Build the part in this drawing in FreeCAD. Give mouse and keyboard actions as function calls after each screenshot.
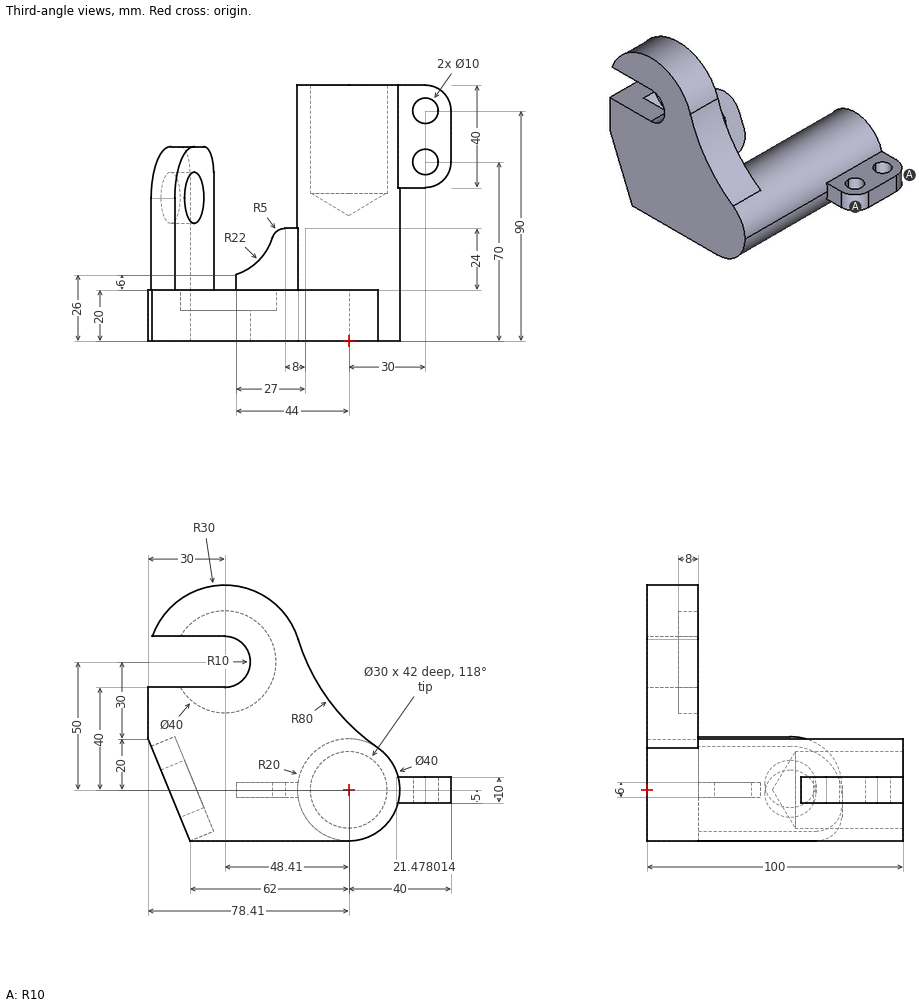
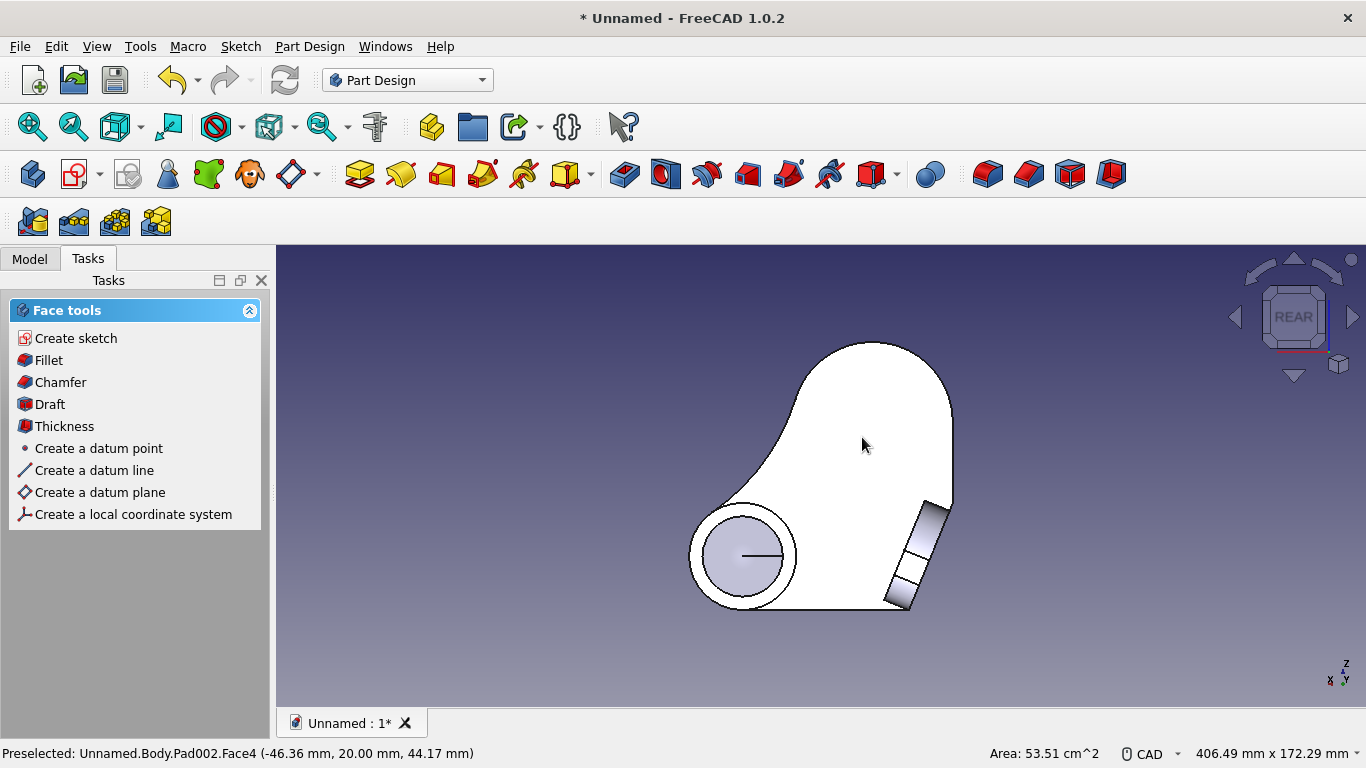
click(74, 174)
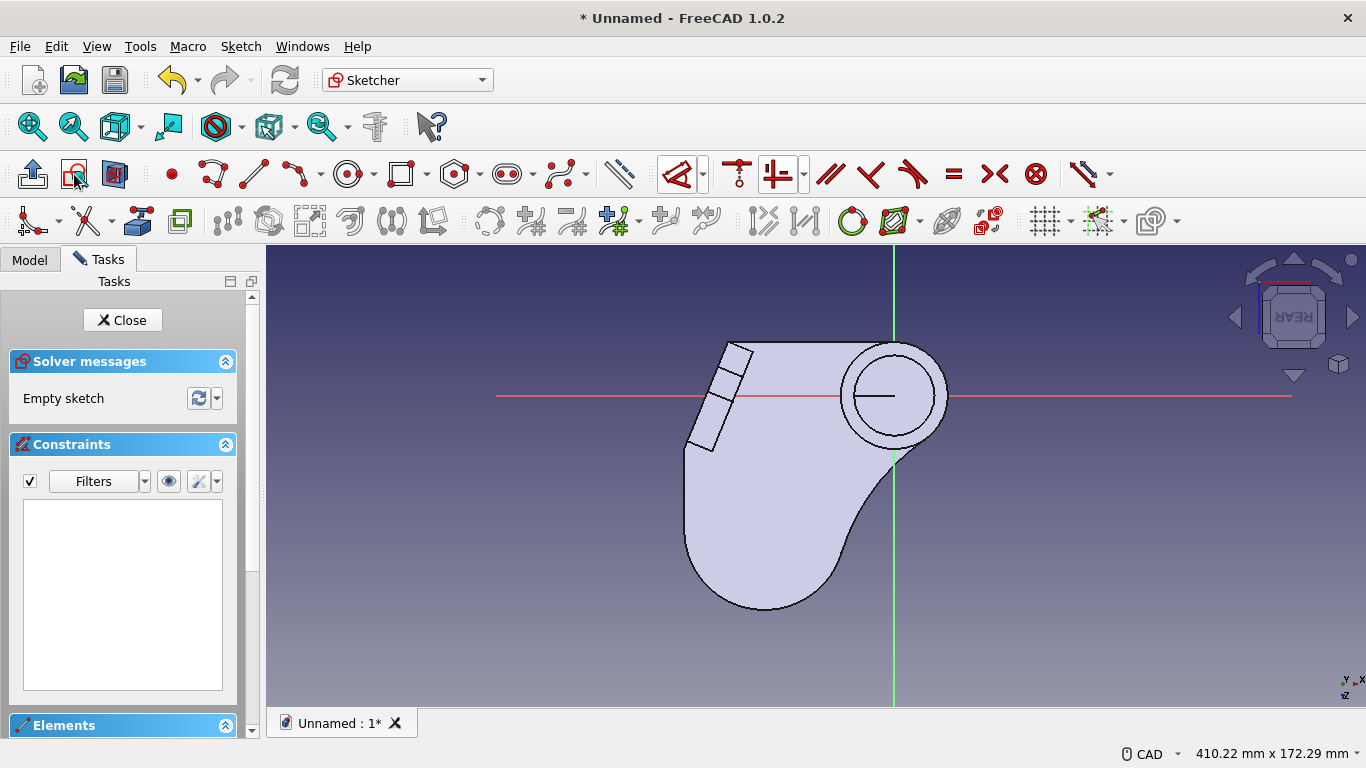
scroll(840, 476, up, 3)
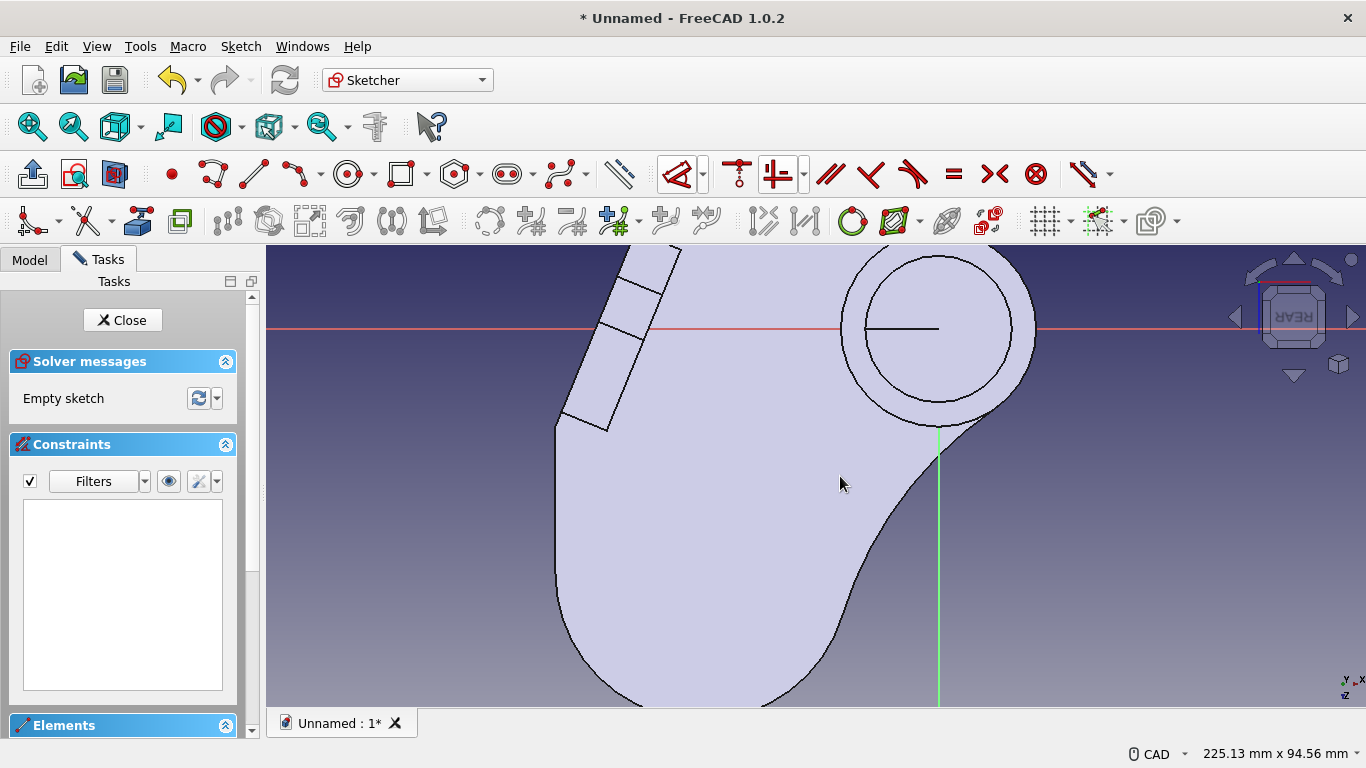
key(g)
key(m)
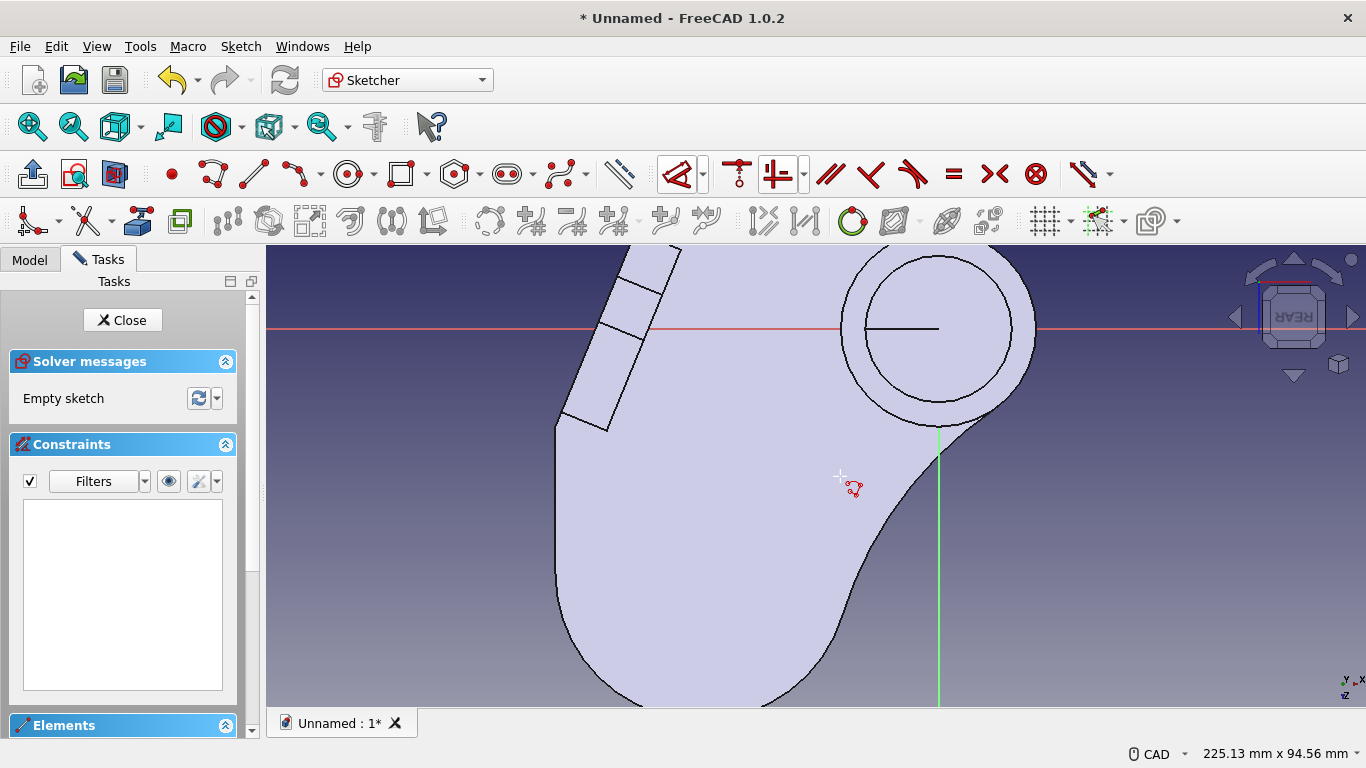
click(702, 524)
click(555, 524)
click(555, 622)
click(702, 622)
right_click(702, 622)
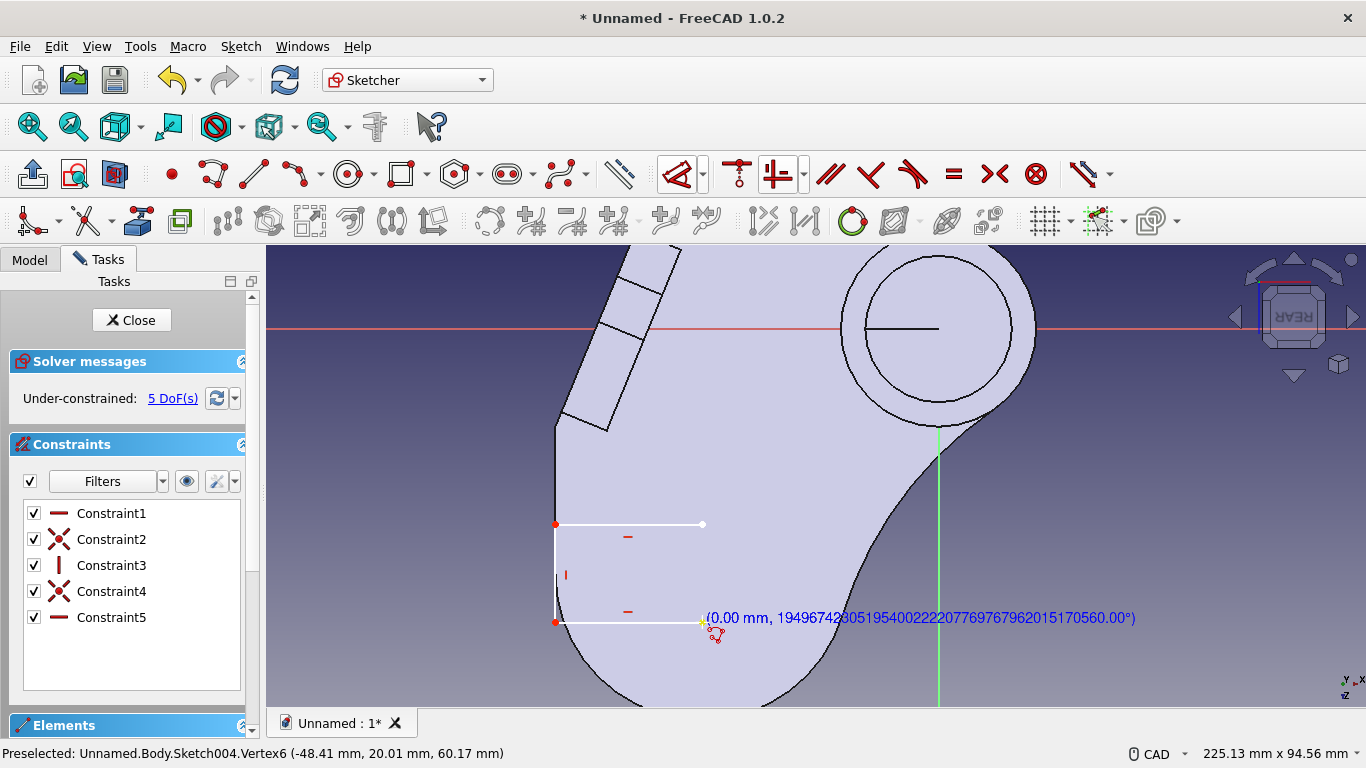
key(g)
key(3)
key(a)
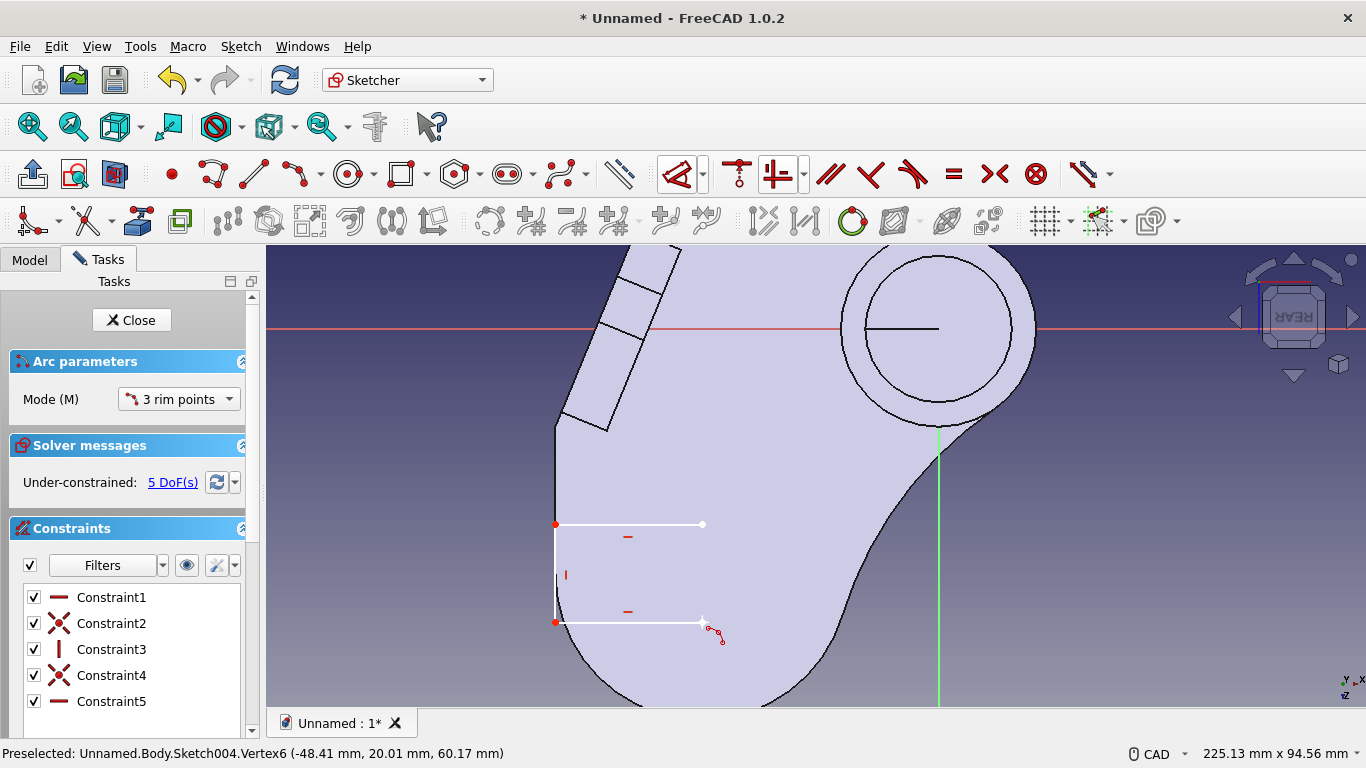
click(702, 623)
click(702, 525)
click(751, 573)
key(Escape)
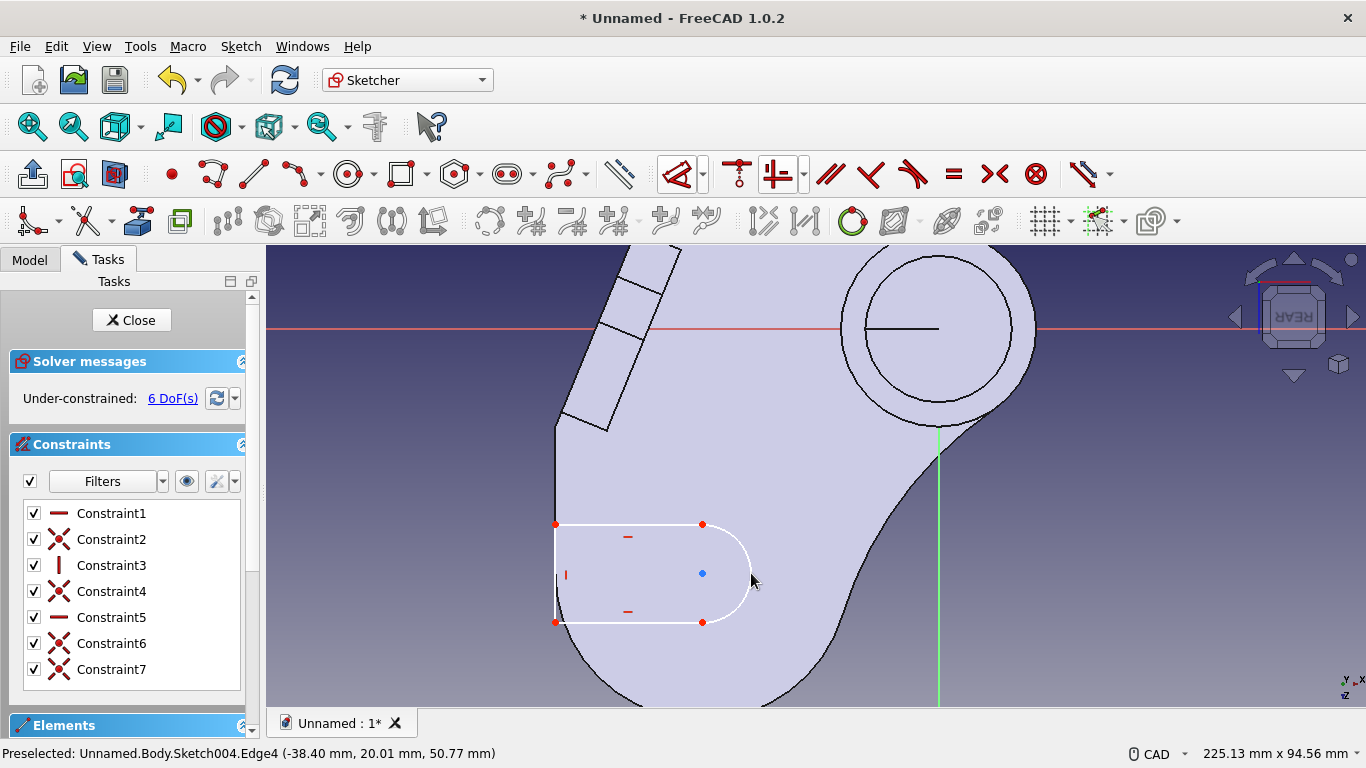
click(658, 525)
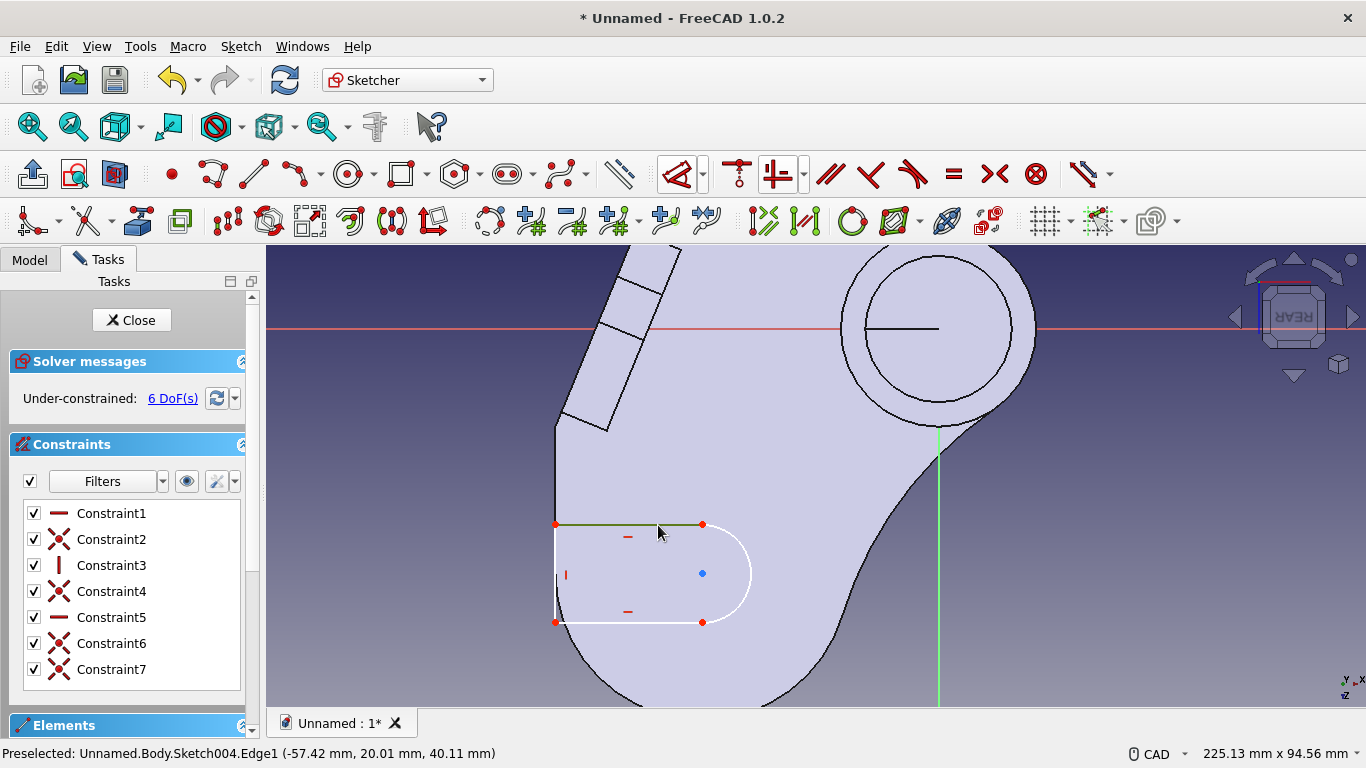
click(742, 603)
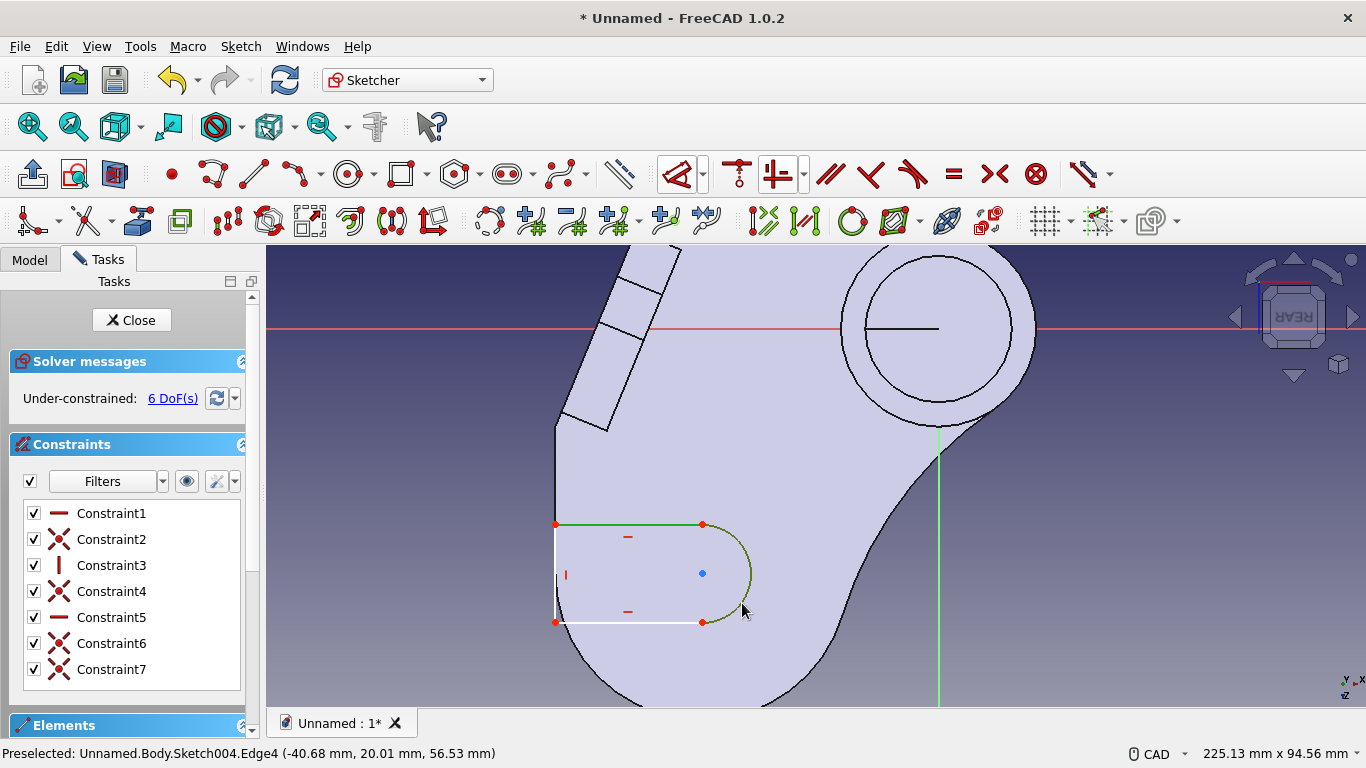
key(t)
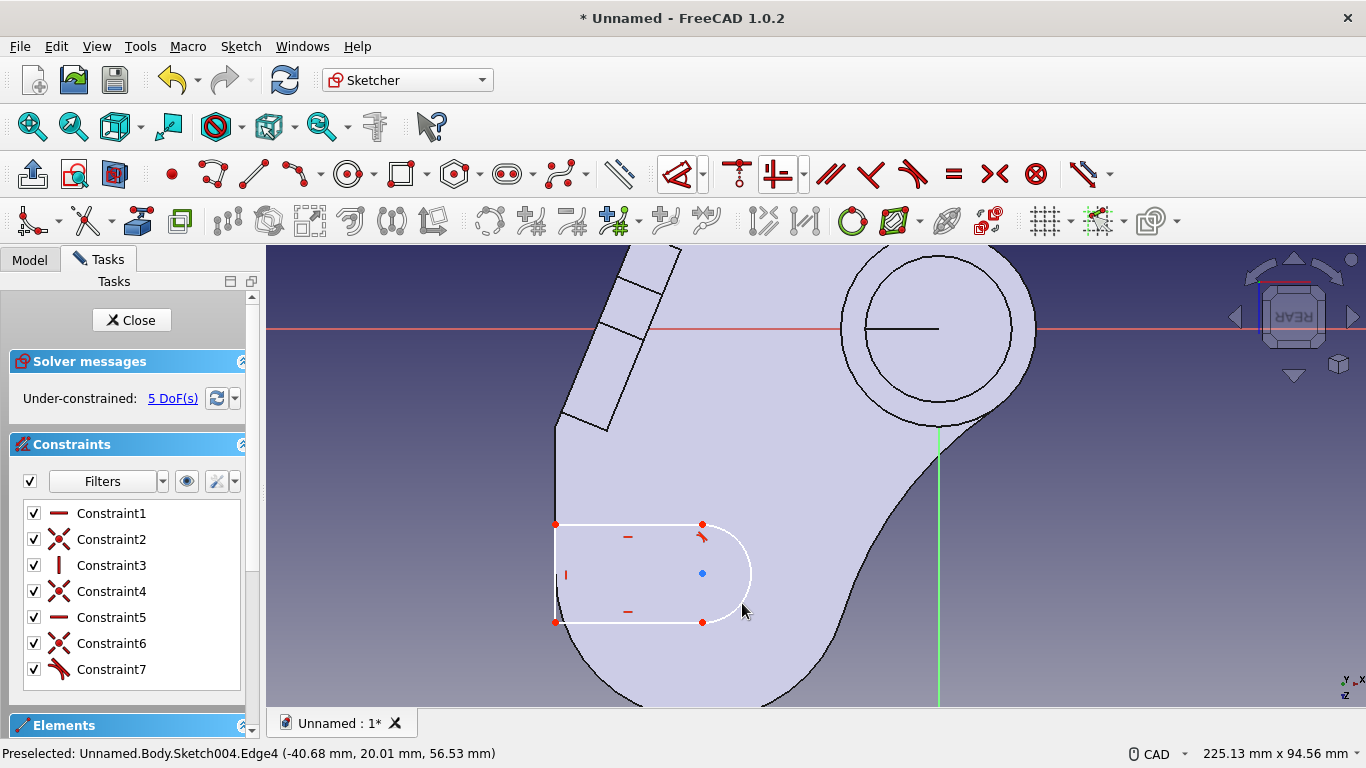
click(599, 623)